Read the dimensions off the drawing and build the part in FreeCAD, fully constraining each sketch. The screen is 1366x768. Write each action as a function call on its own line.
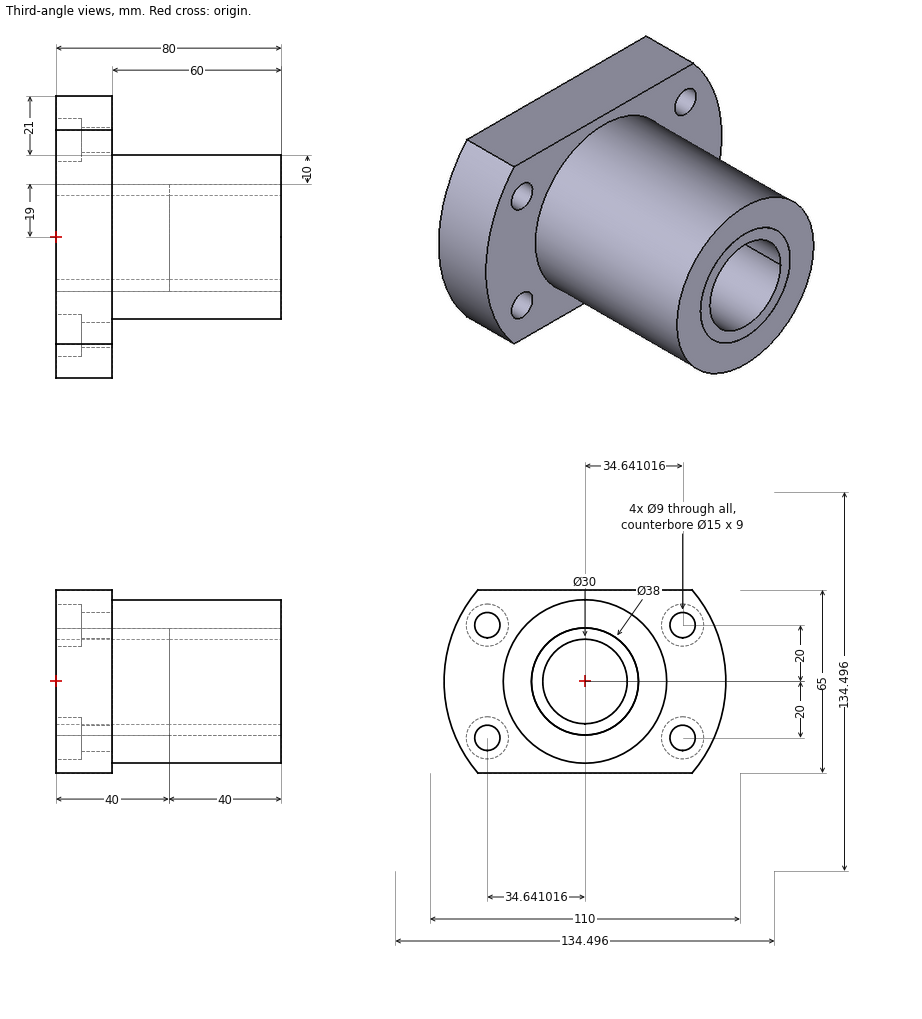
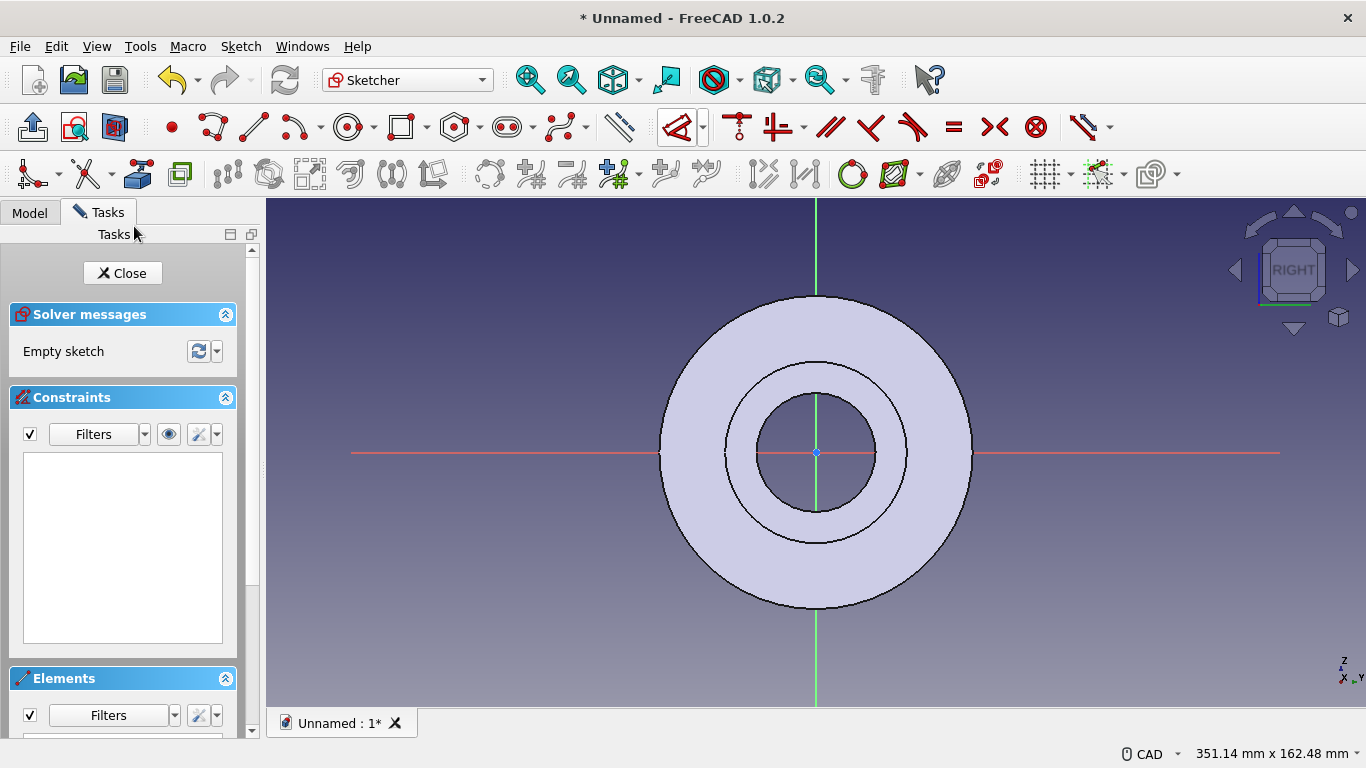
click(115, 128)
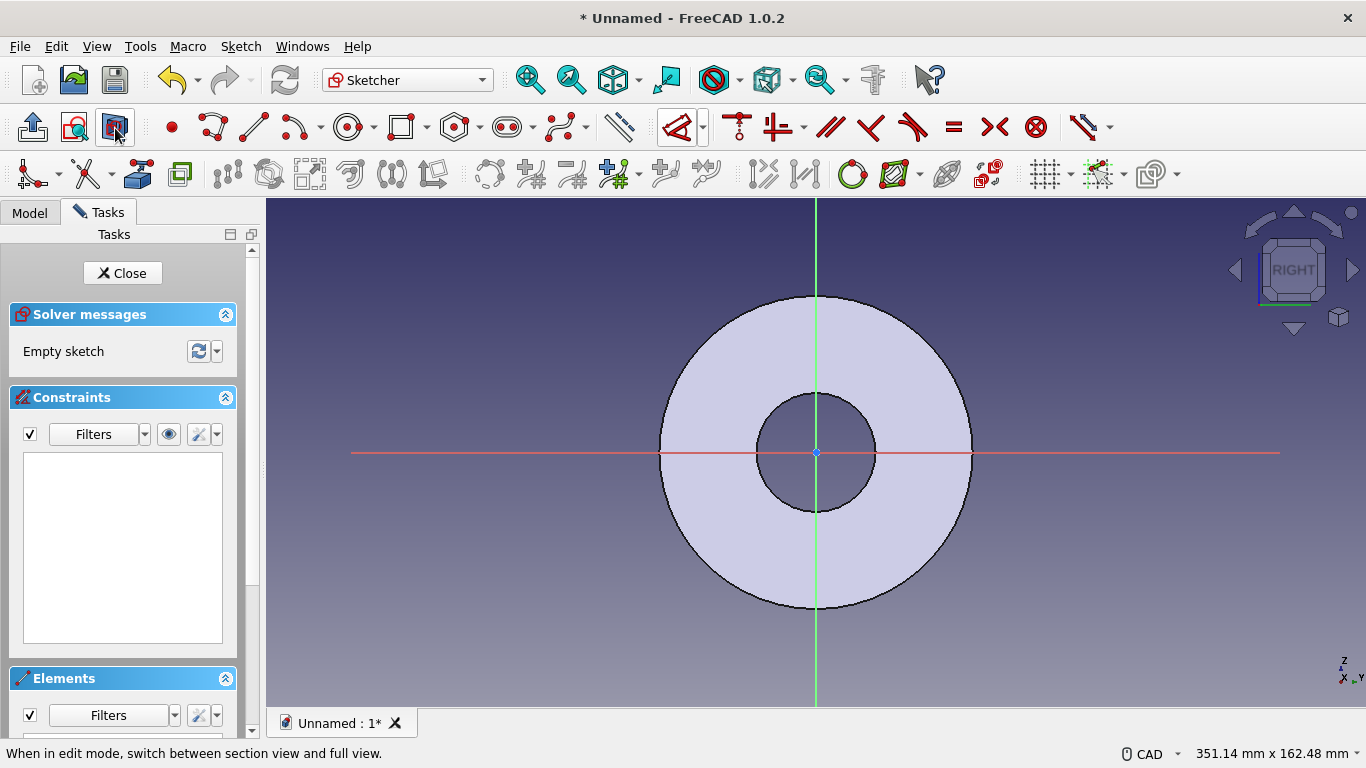
scroll(872, 452, up, 4)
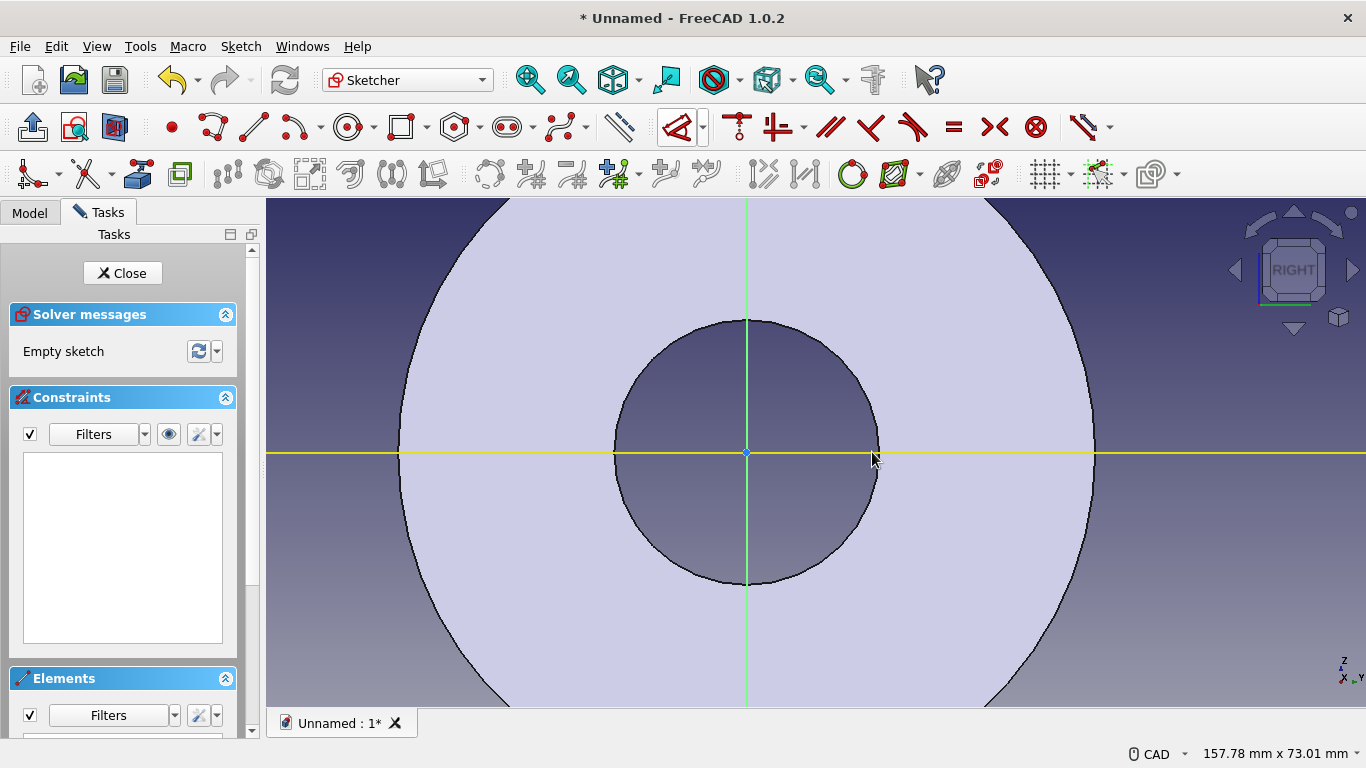
click(348, 128)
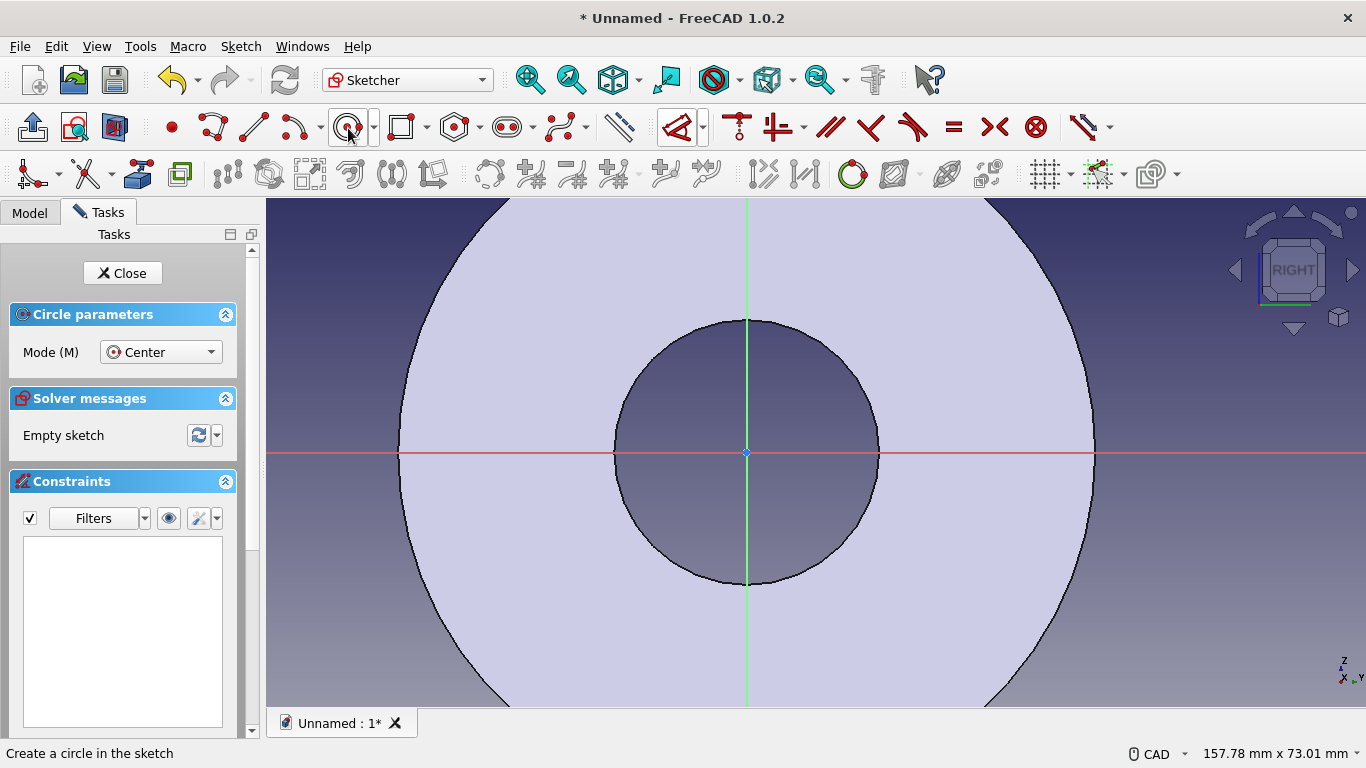
click(988, 313)
click(1010, 291)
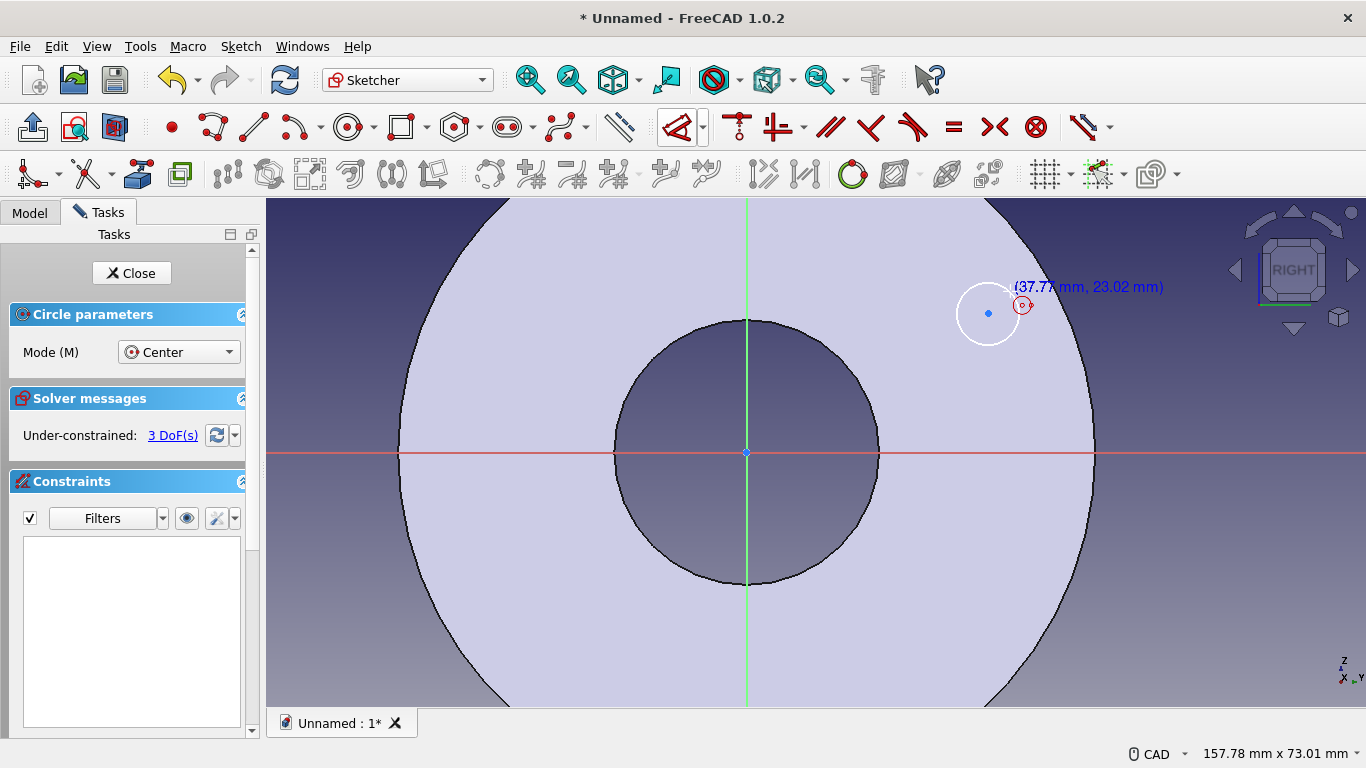
click(988, 592)
click(1010, 570)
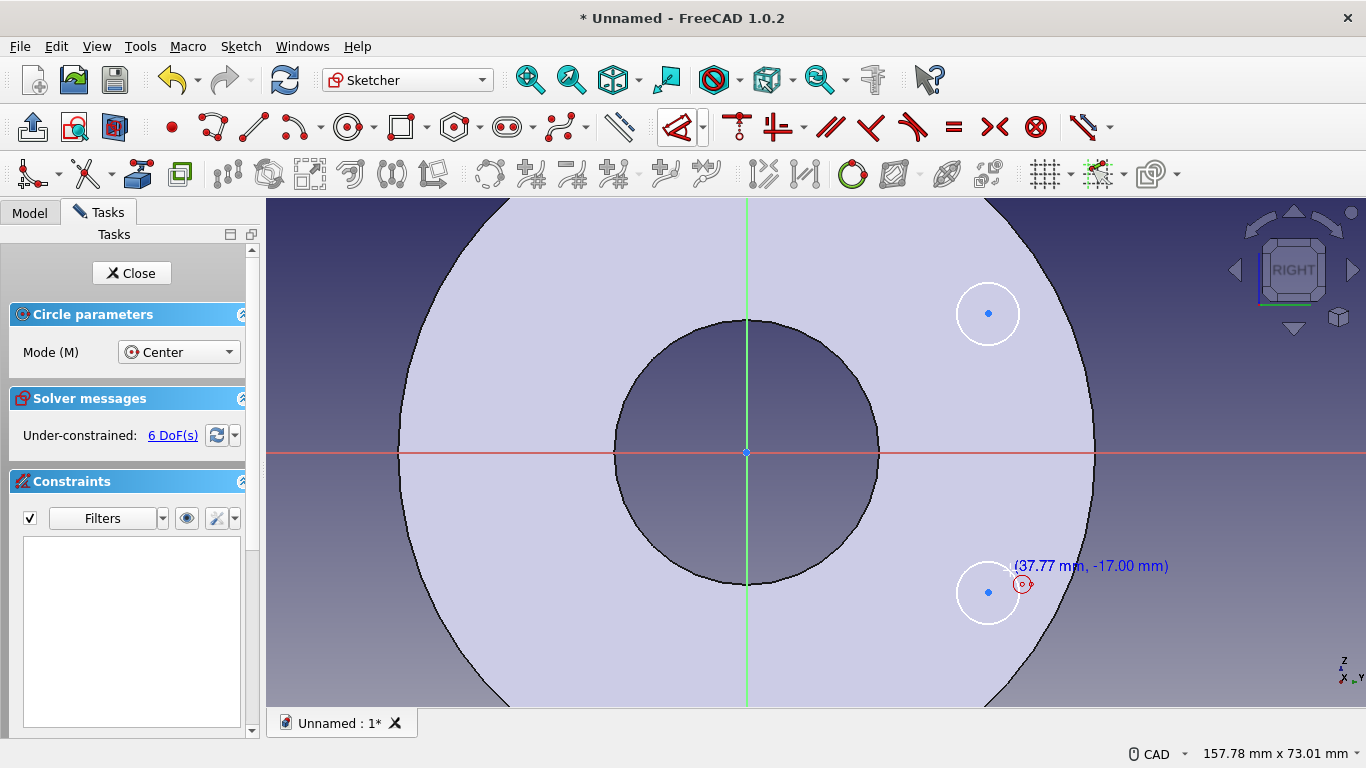
click(505, 592)
click(527, 570)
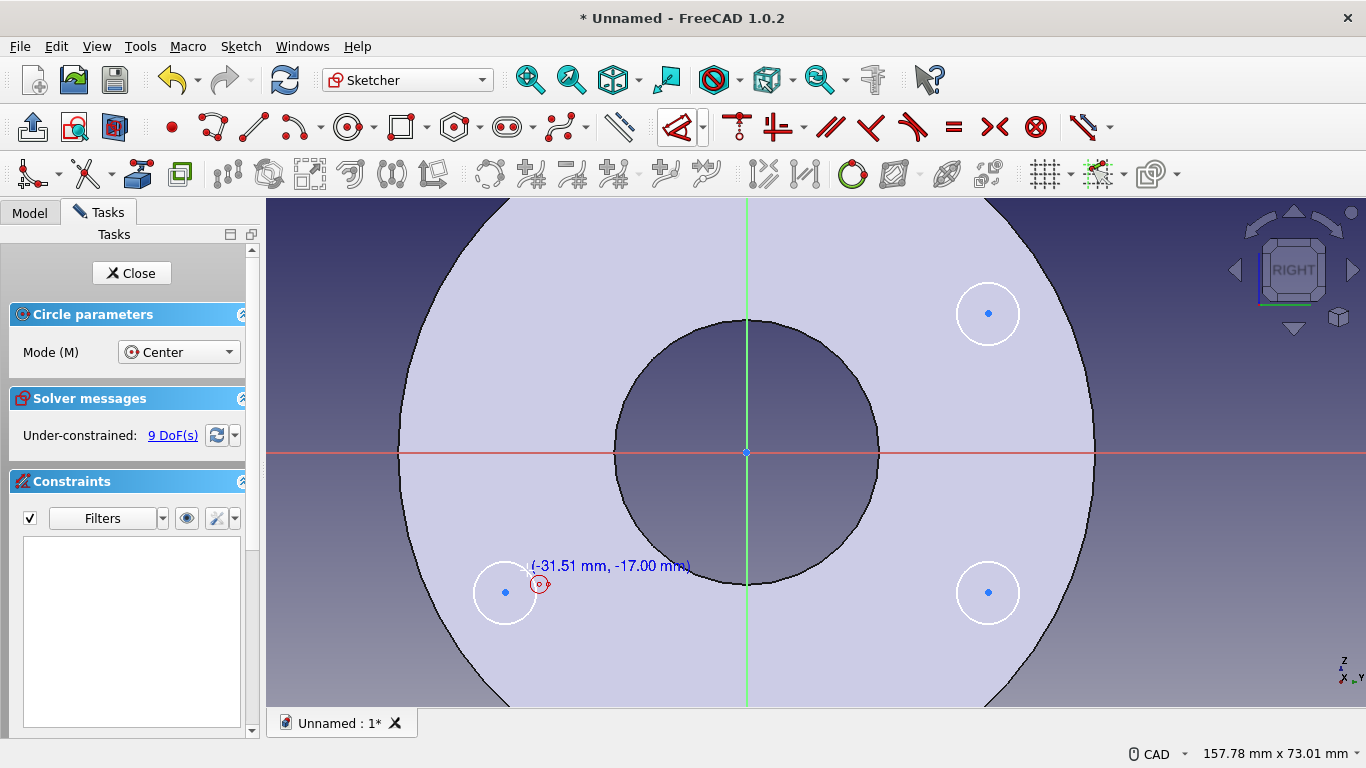
click(505, 313)
click(527, 291)
key(Escape)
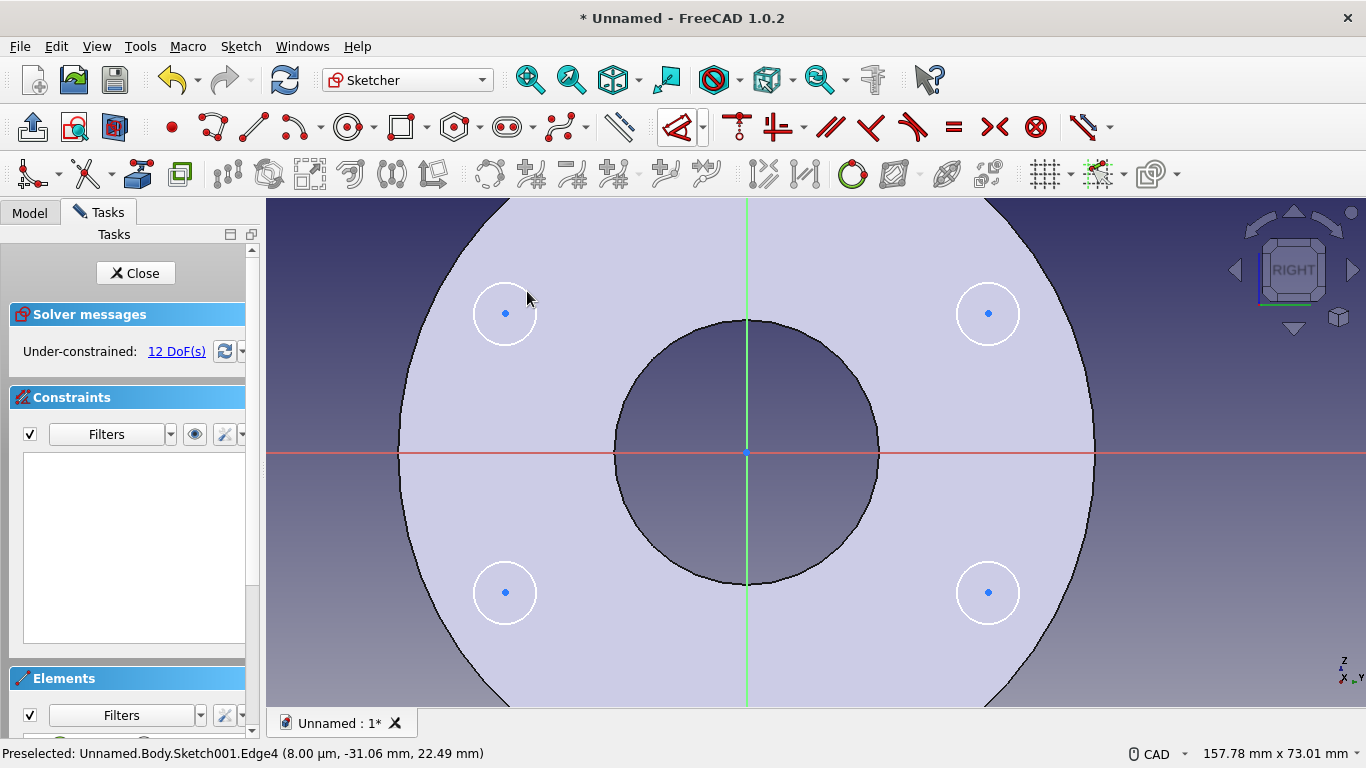
click(1010, 292)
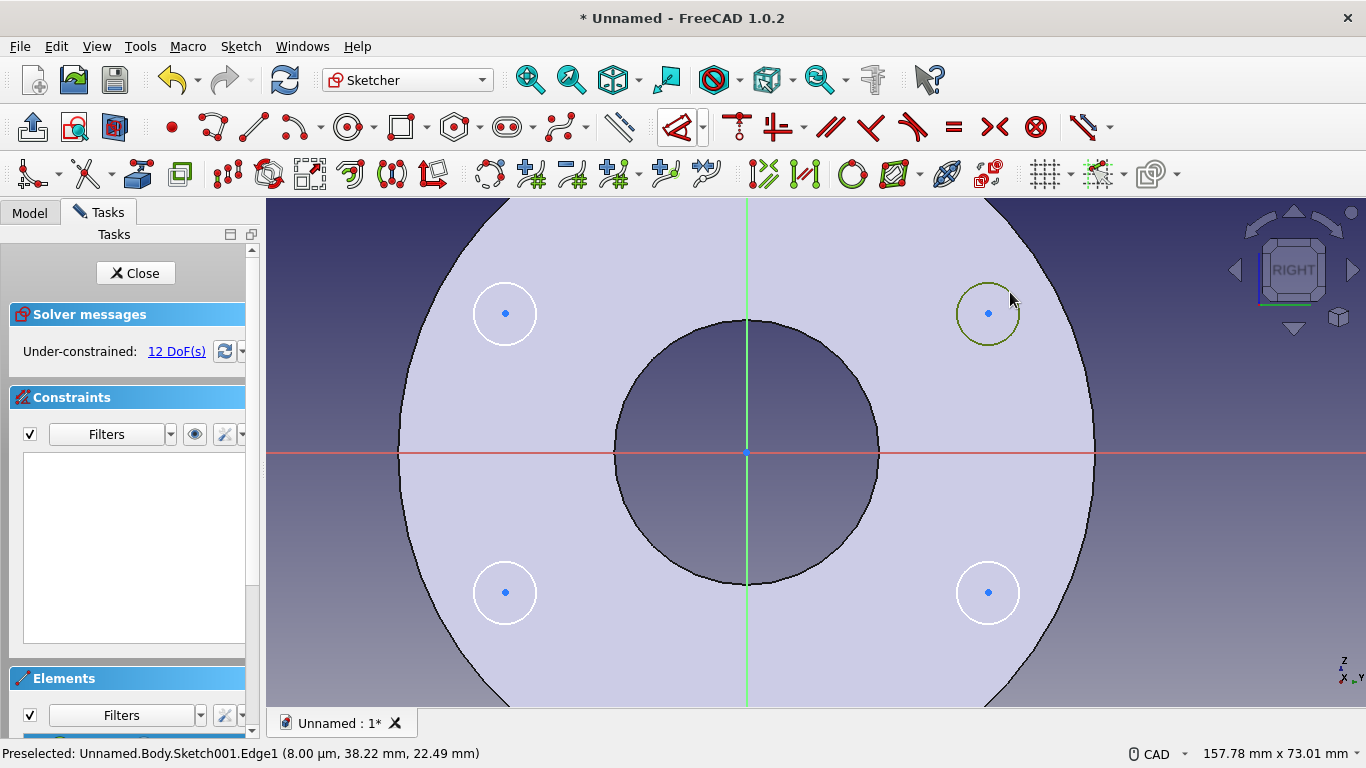
click(1010, 571)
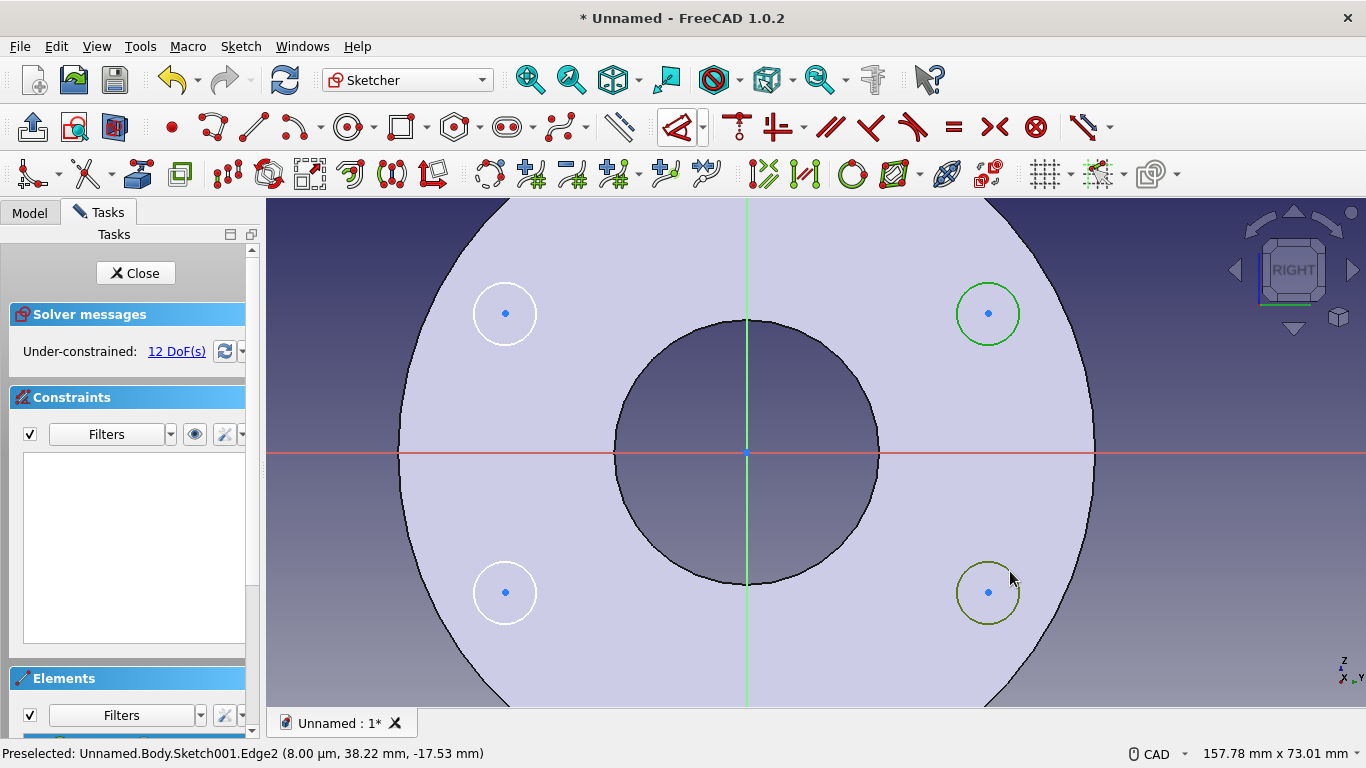
click(527, 571)